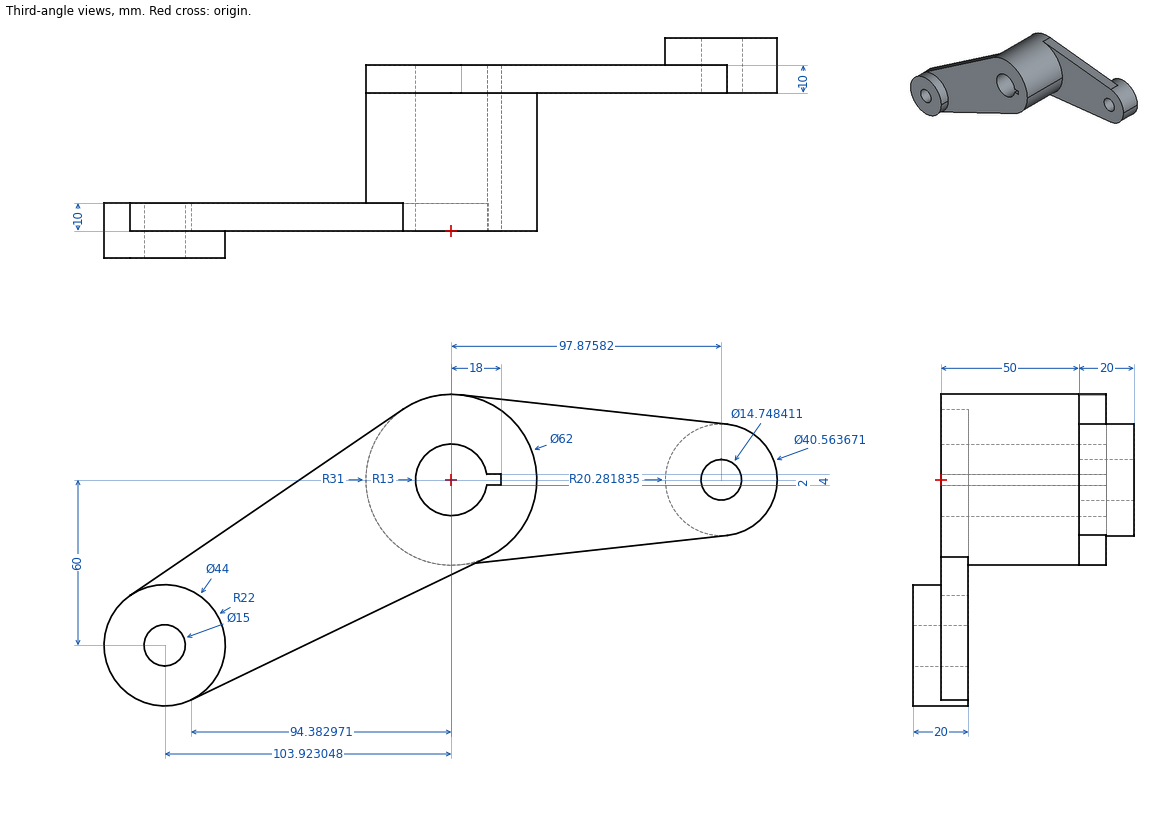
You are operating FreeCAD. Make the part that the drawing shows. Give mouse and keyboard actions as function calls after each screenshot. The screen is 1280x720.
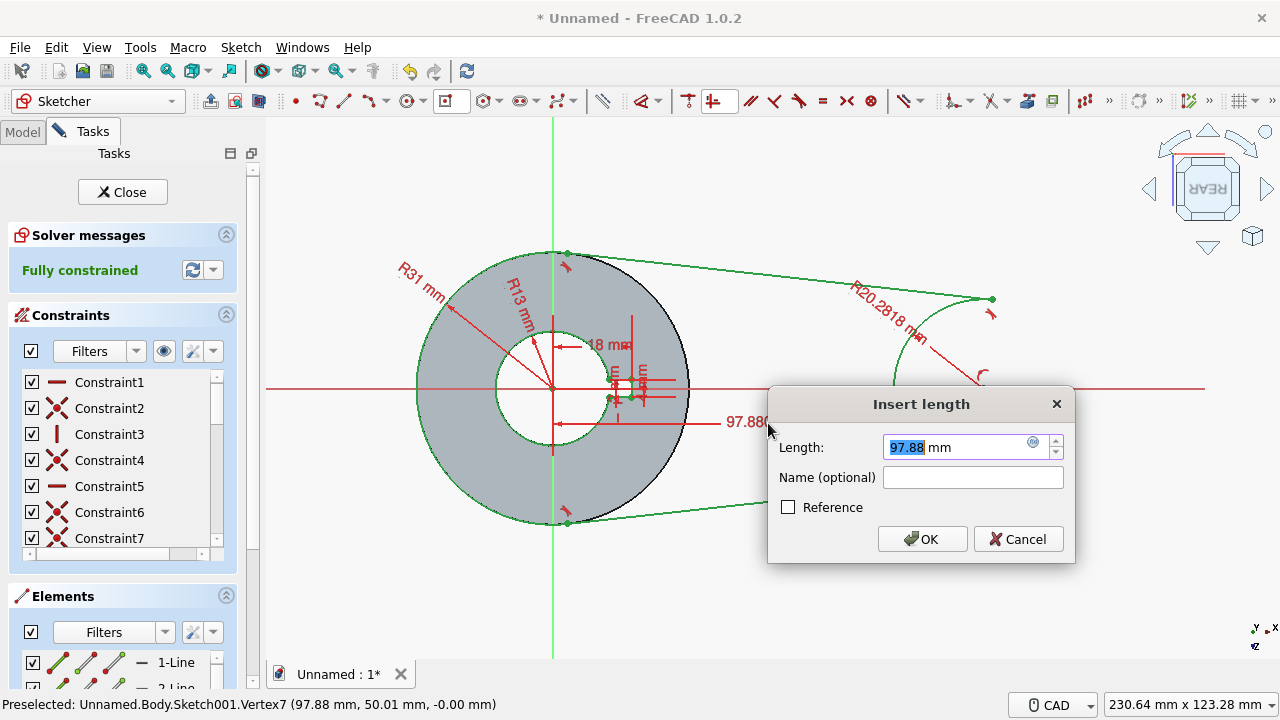
text(97.87582)
key(Return)
key(Escape)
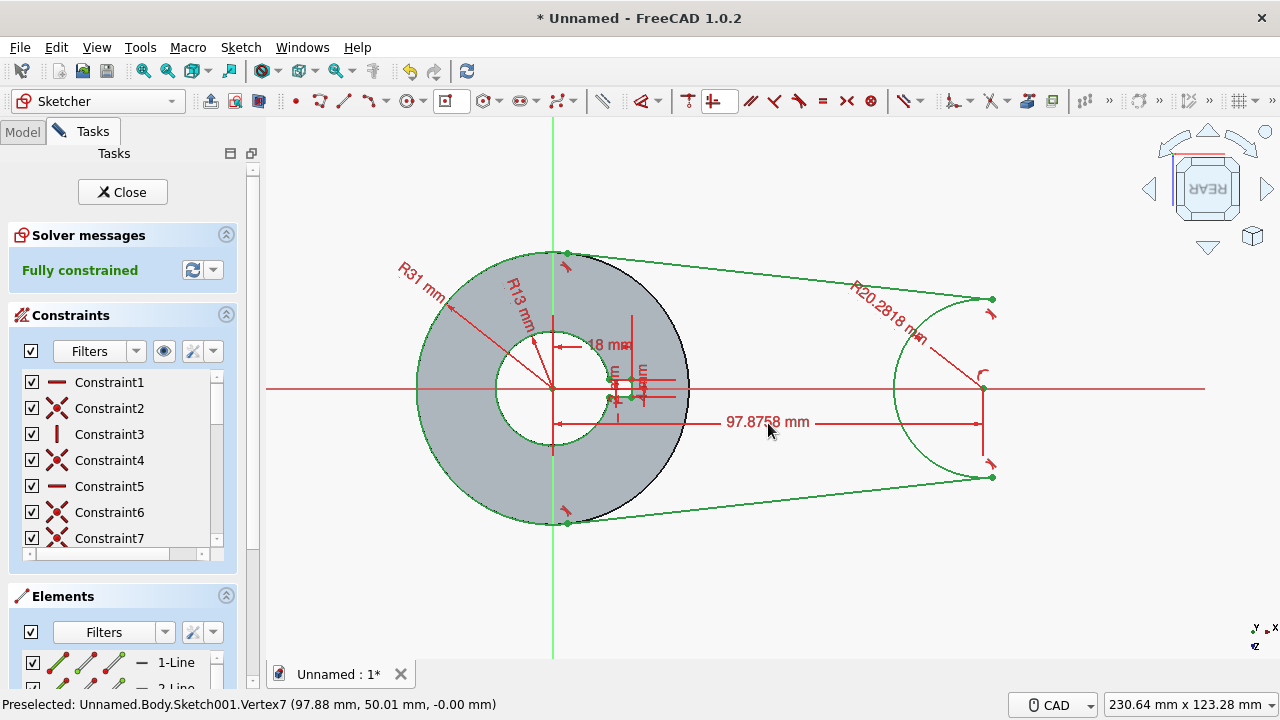
click(123, 192)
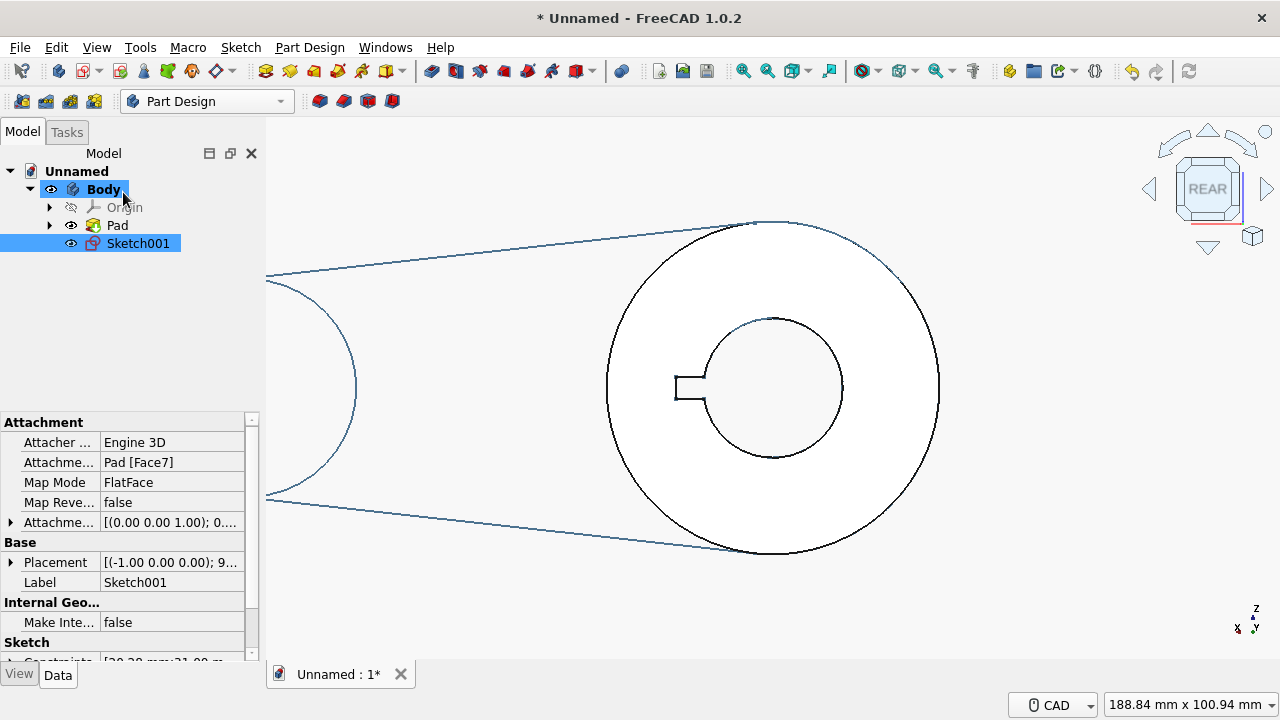
click(266, 72)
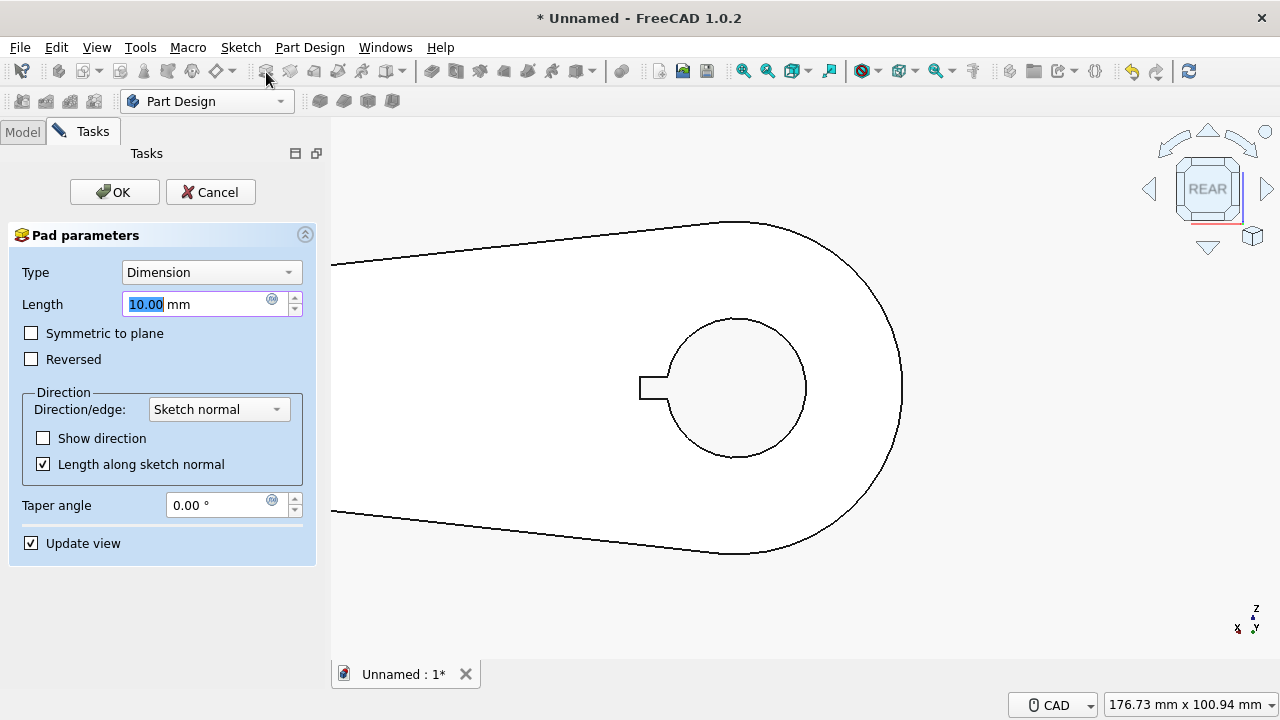
text(10)
key(Tab)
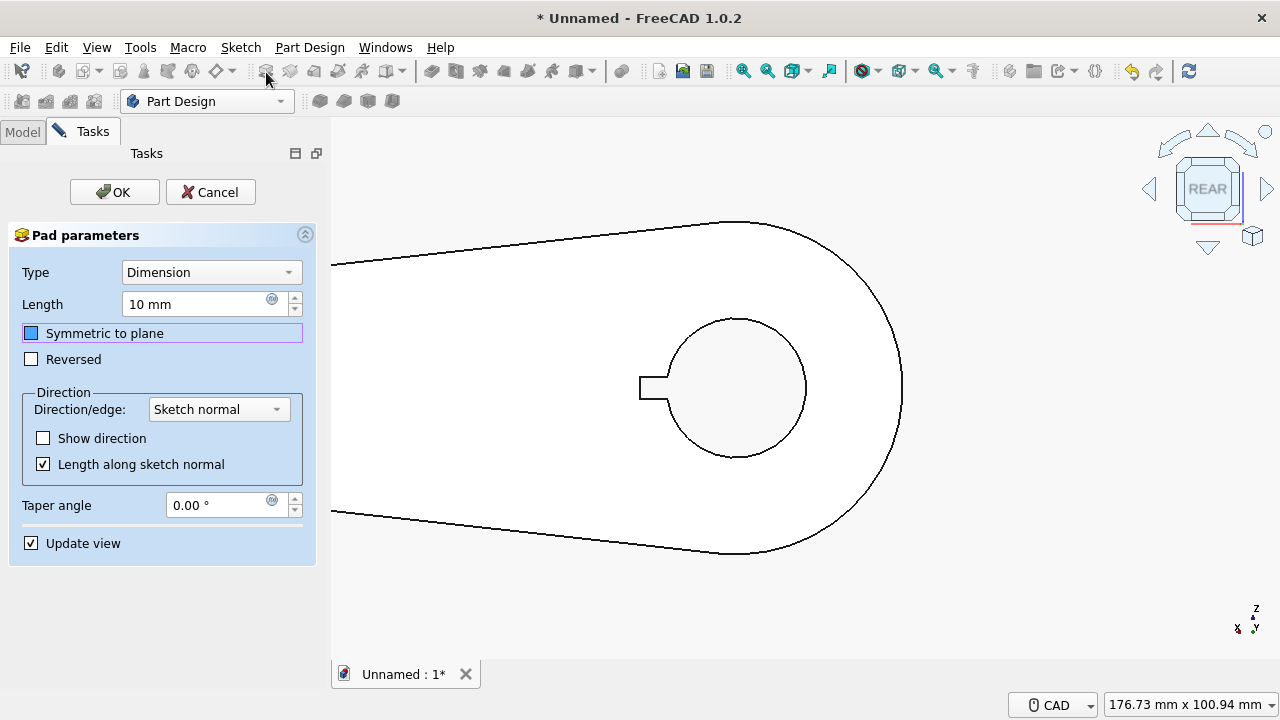
click(115, 192)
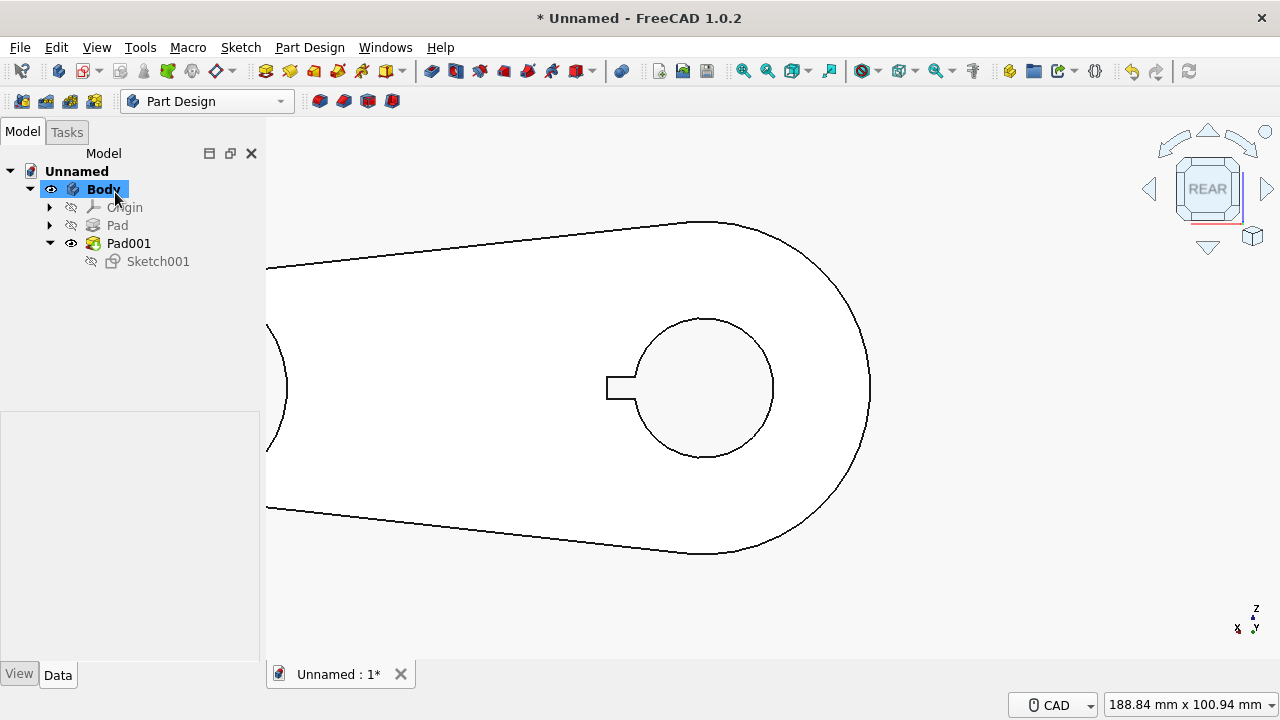
click(744, 72)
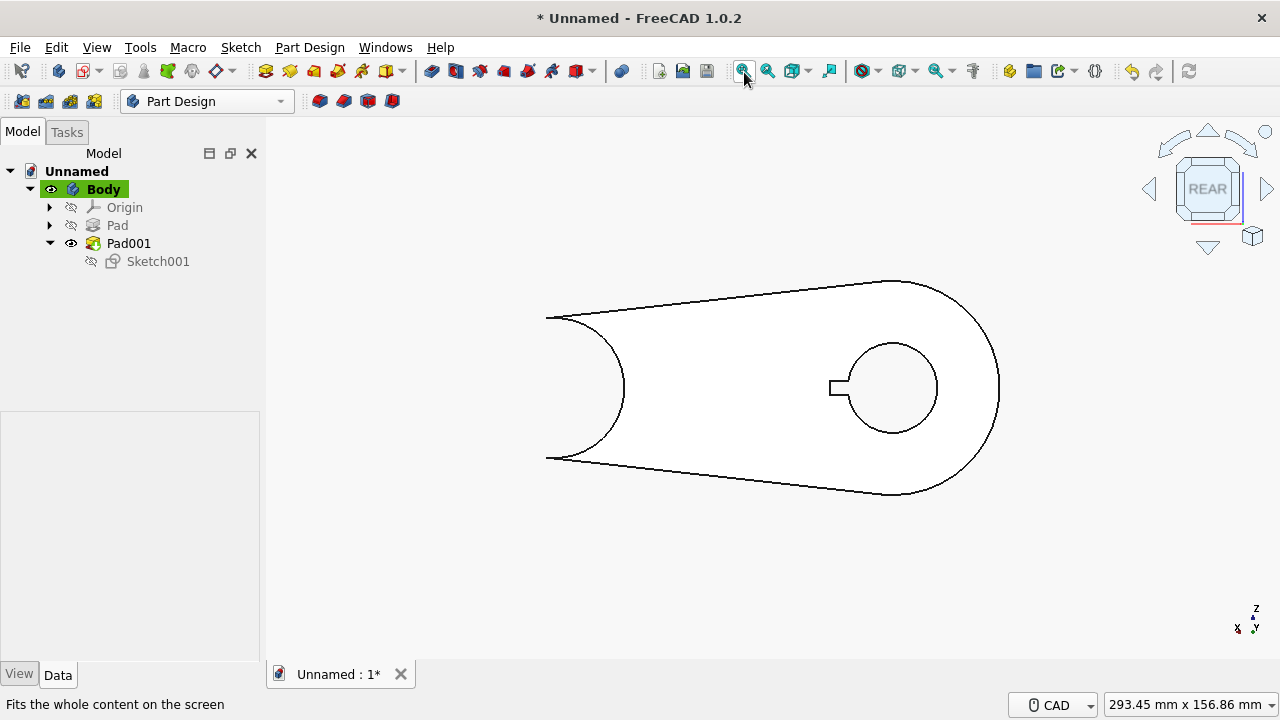
key(0)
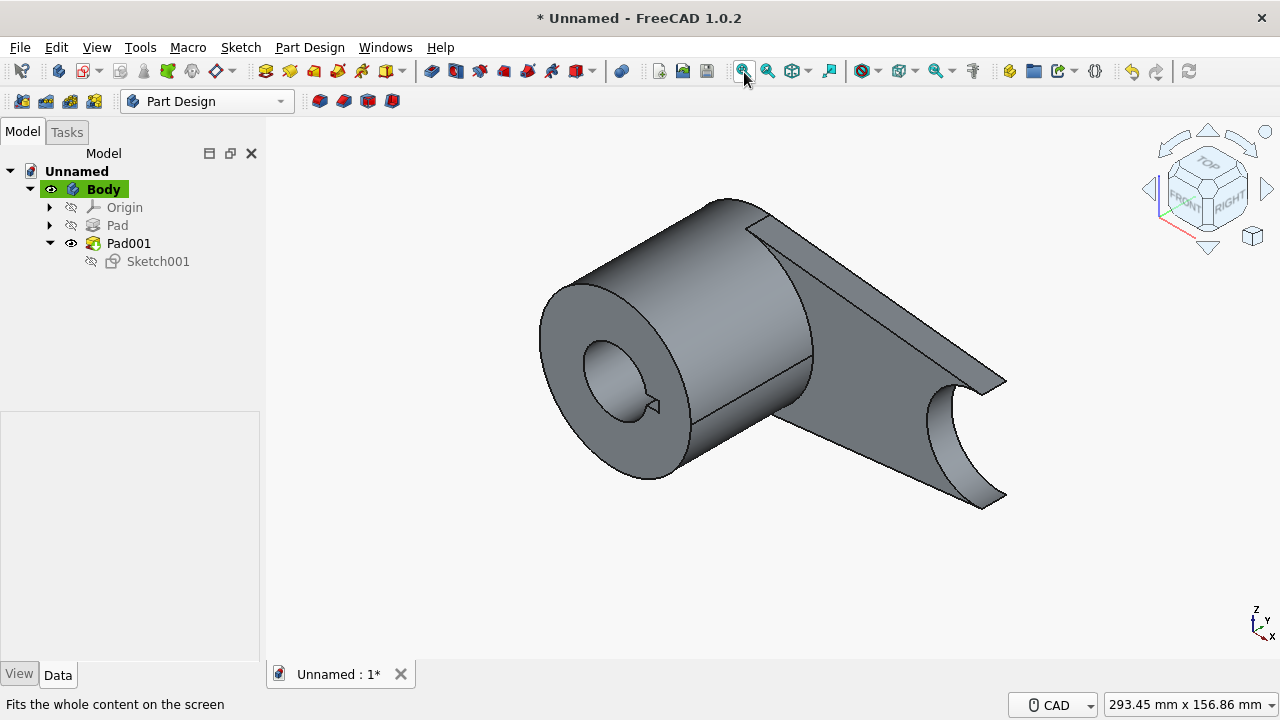
click(864, 383)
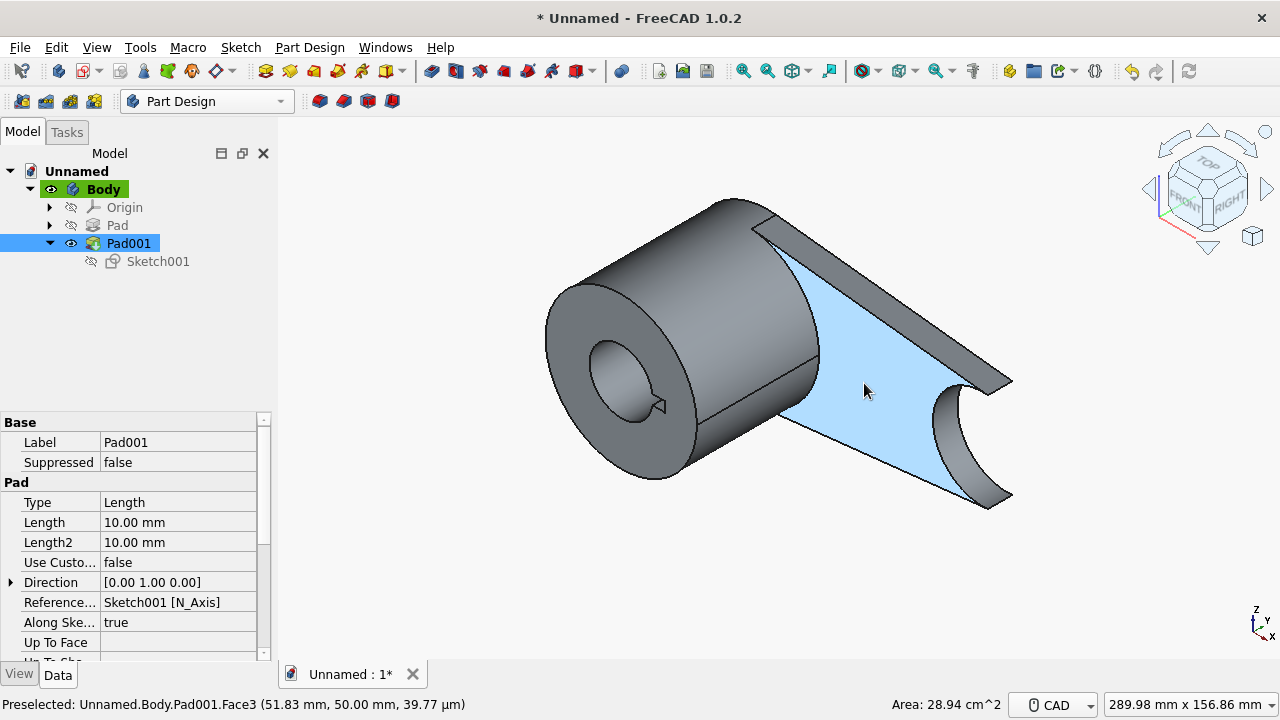
click(84, 72)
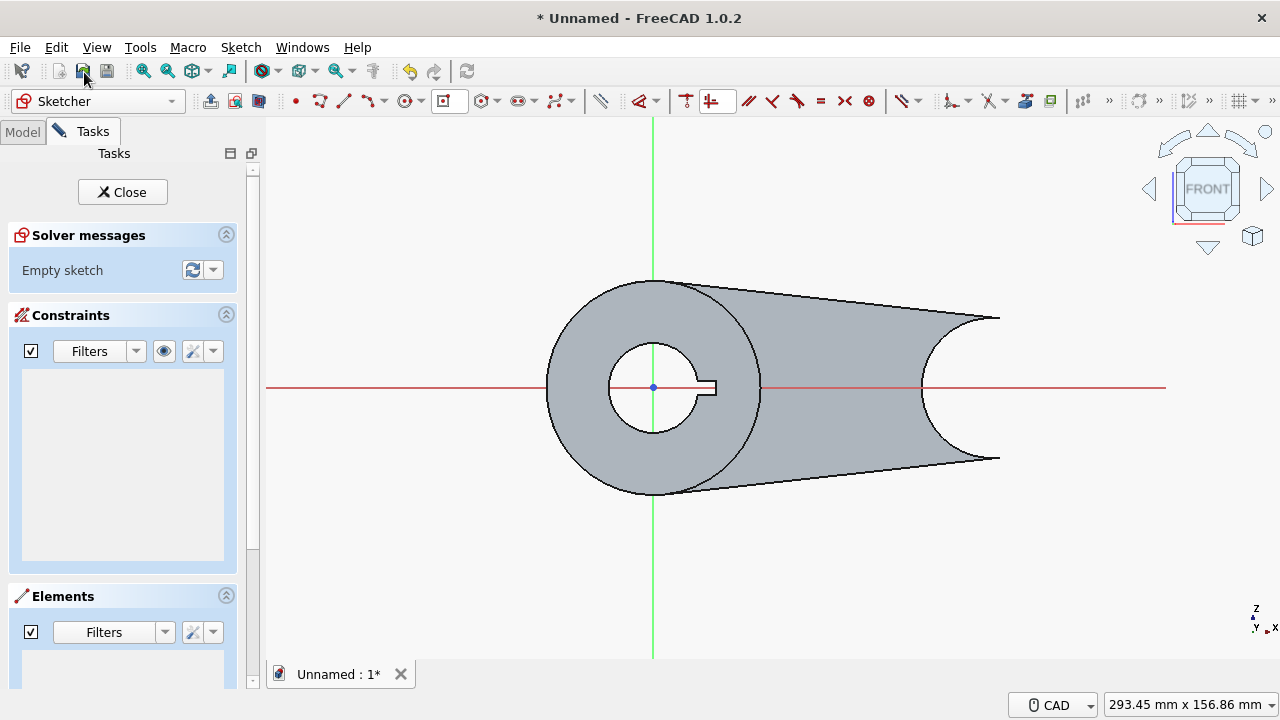
click(260, 102)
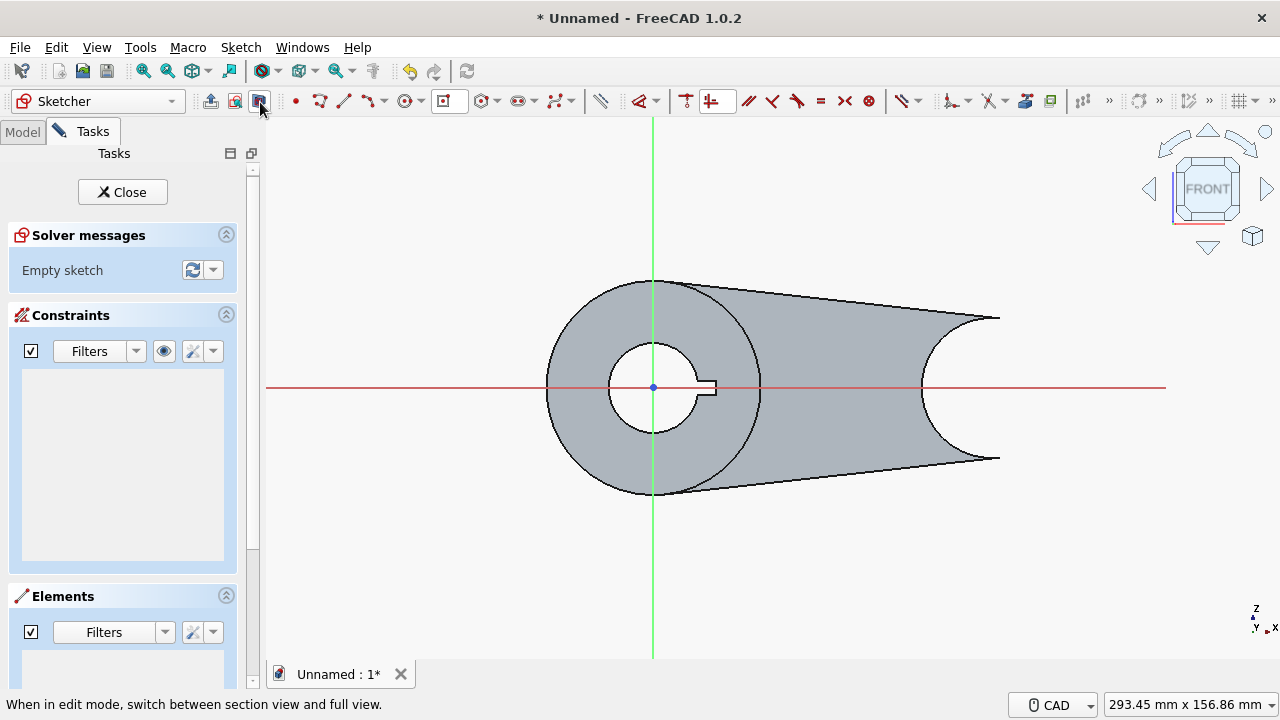
scroll(1115, 388, up, 4)